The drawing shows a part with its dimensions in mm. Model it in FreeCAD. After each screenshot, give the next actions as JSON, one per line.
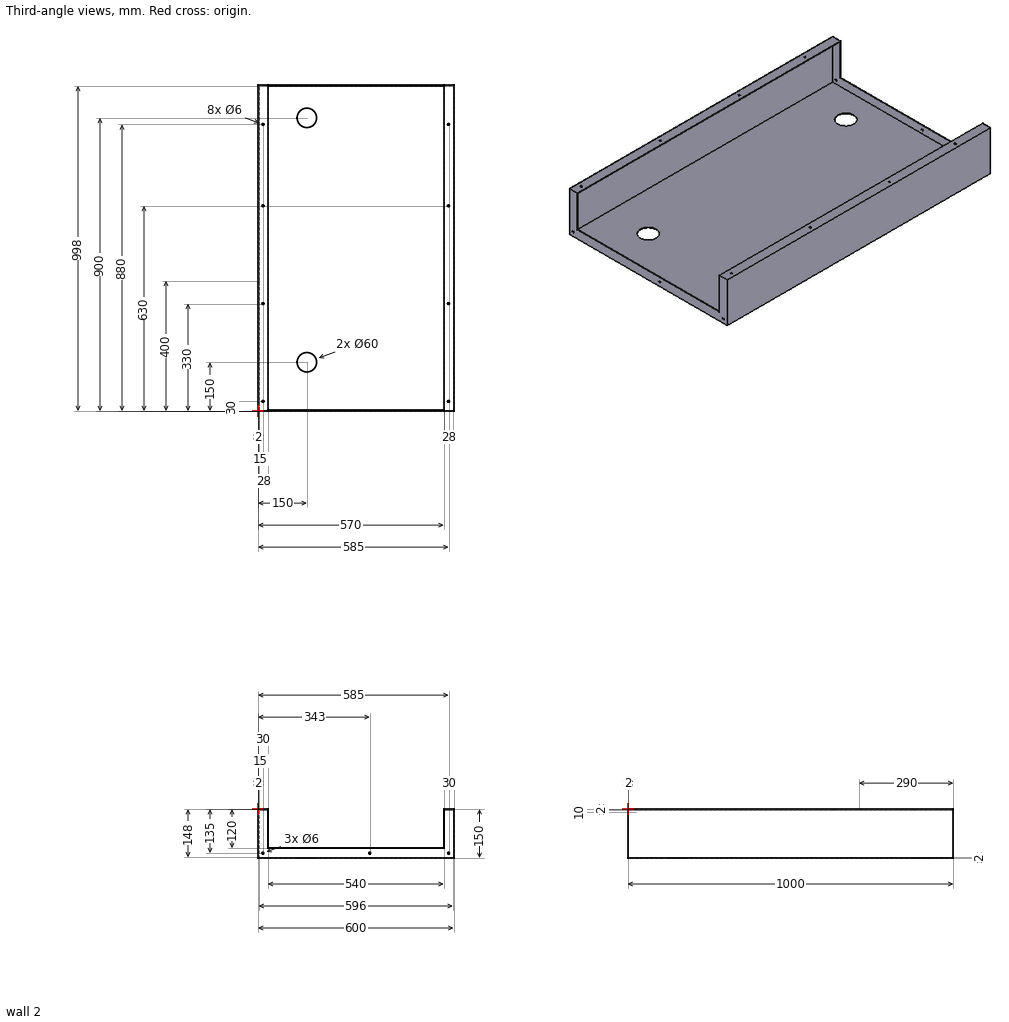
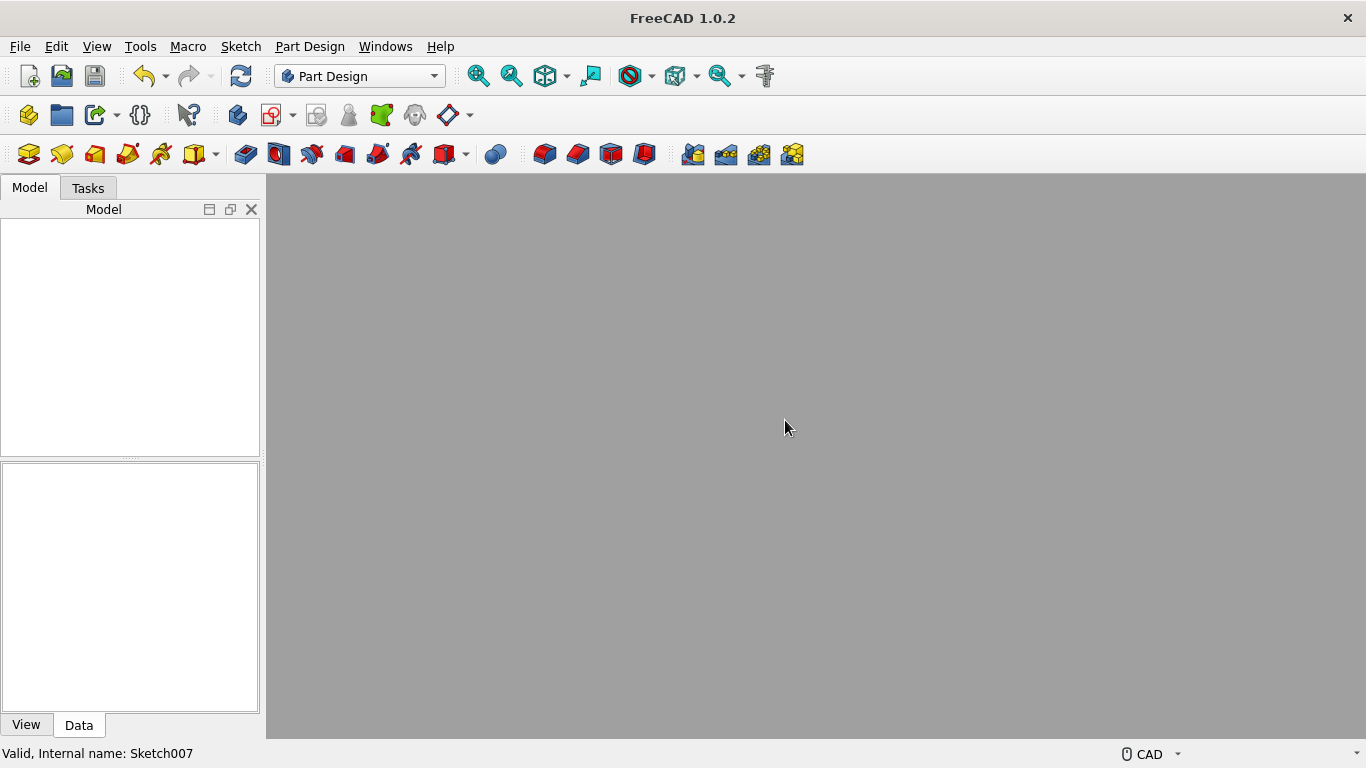
{"action": "left_click", "coordinate": [29, 76]}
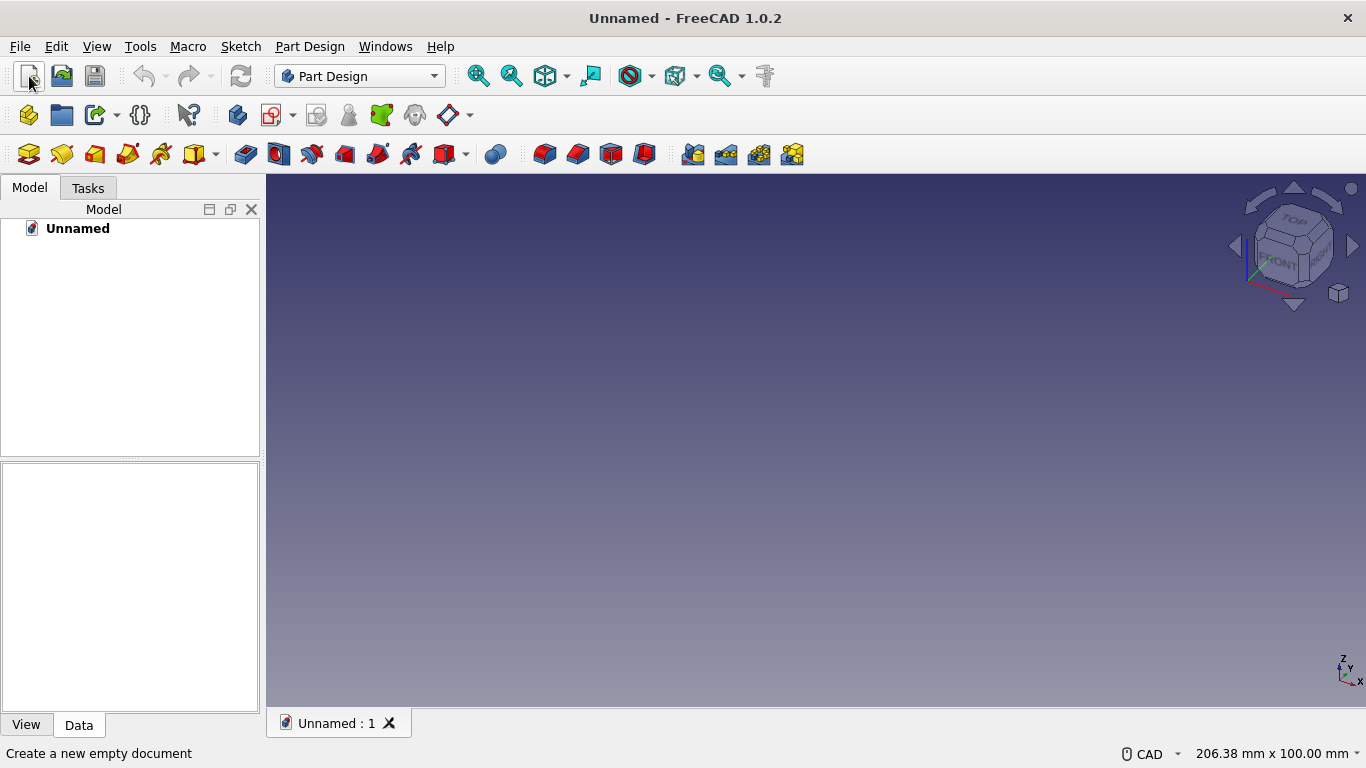
{"action": "left_click", "coordinate": [270, 116]}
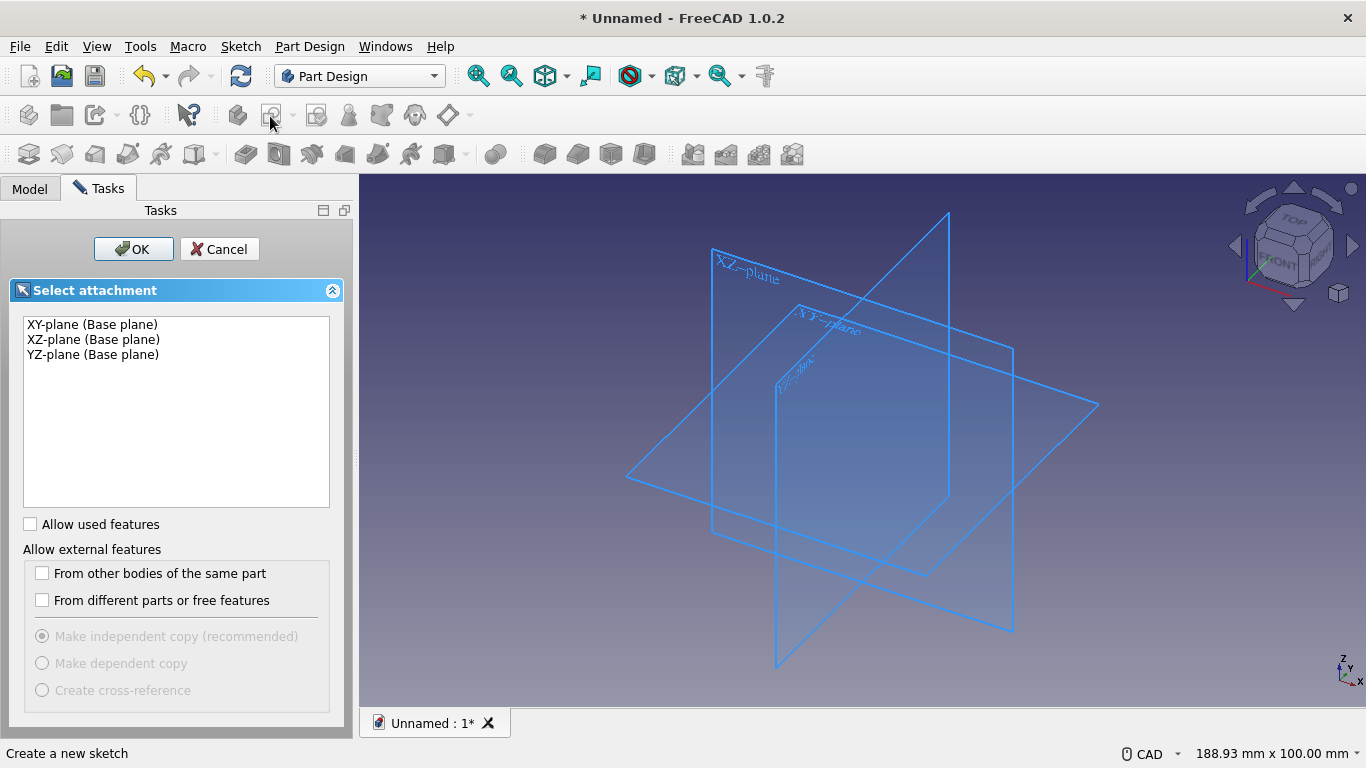
{"action": "left_click", "coordinate": [84, 340]}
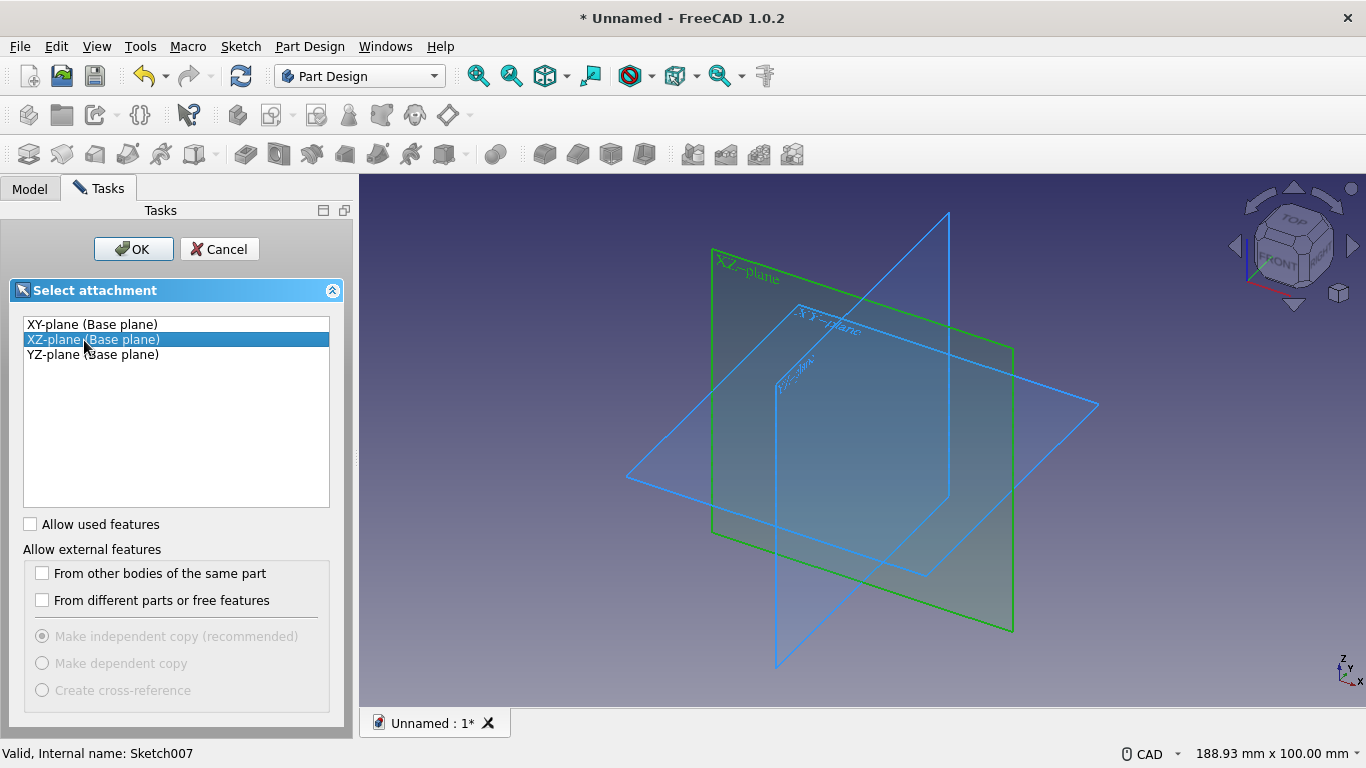
{"action": "left_click", "coordinate": [134, 249]}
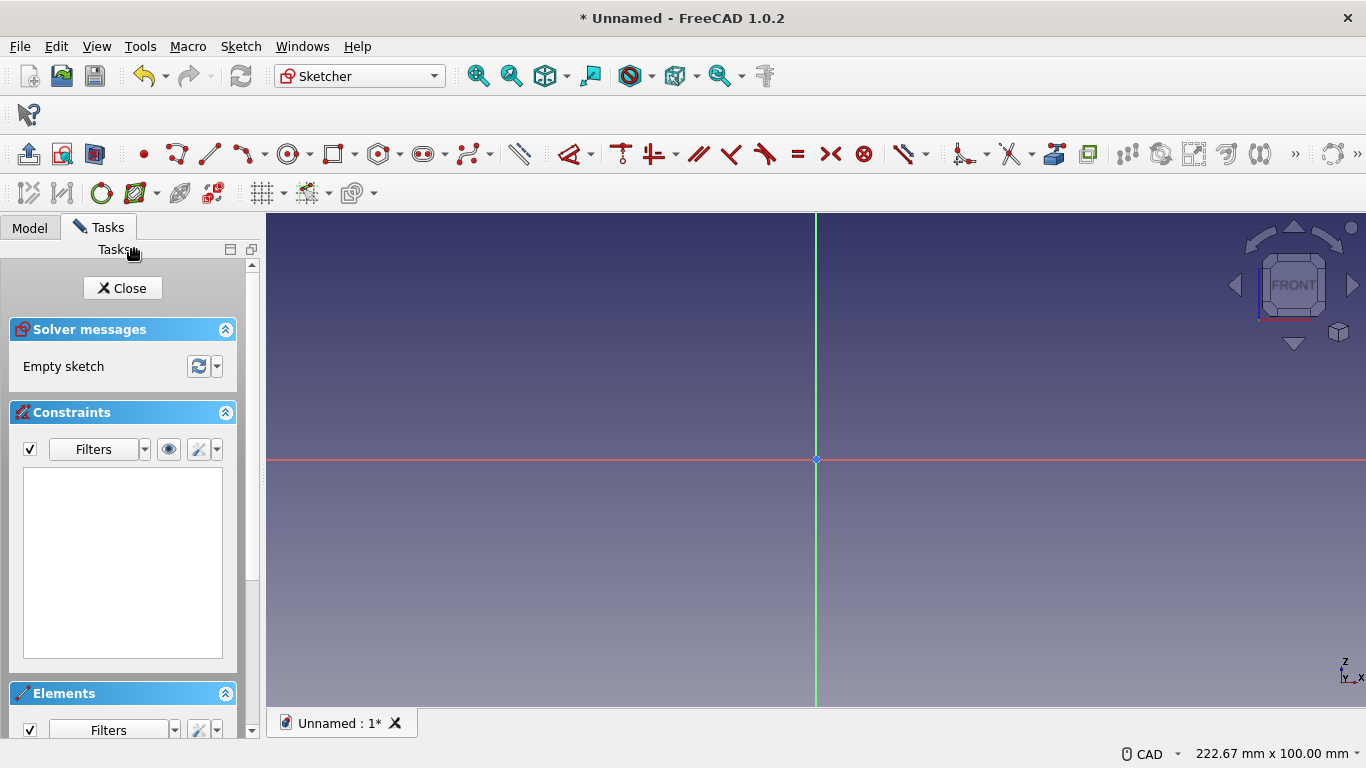
{"action": "scroll", "coordinate": [355, 366], "scroll_direction": "down", "scroll_amount": 8}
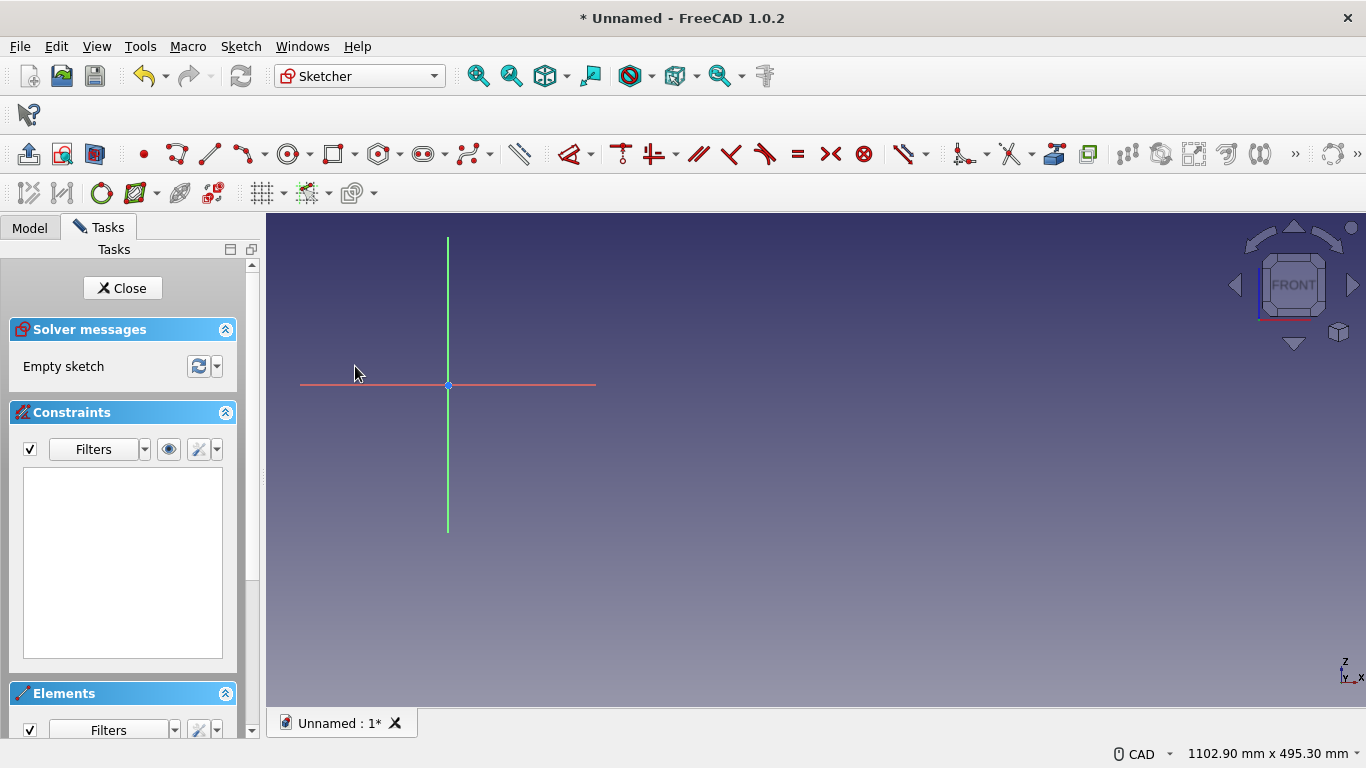
{"action": "left_click", "coordinate": [332, 154]}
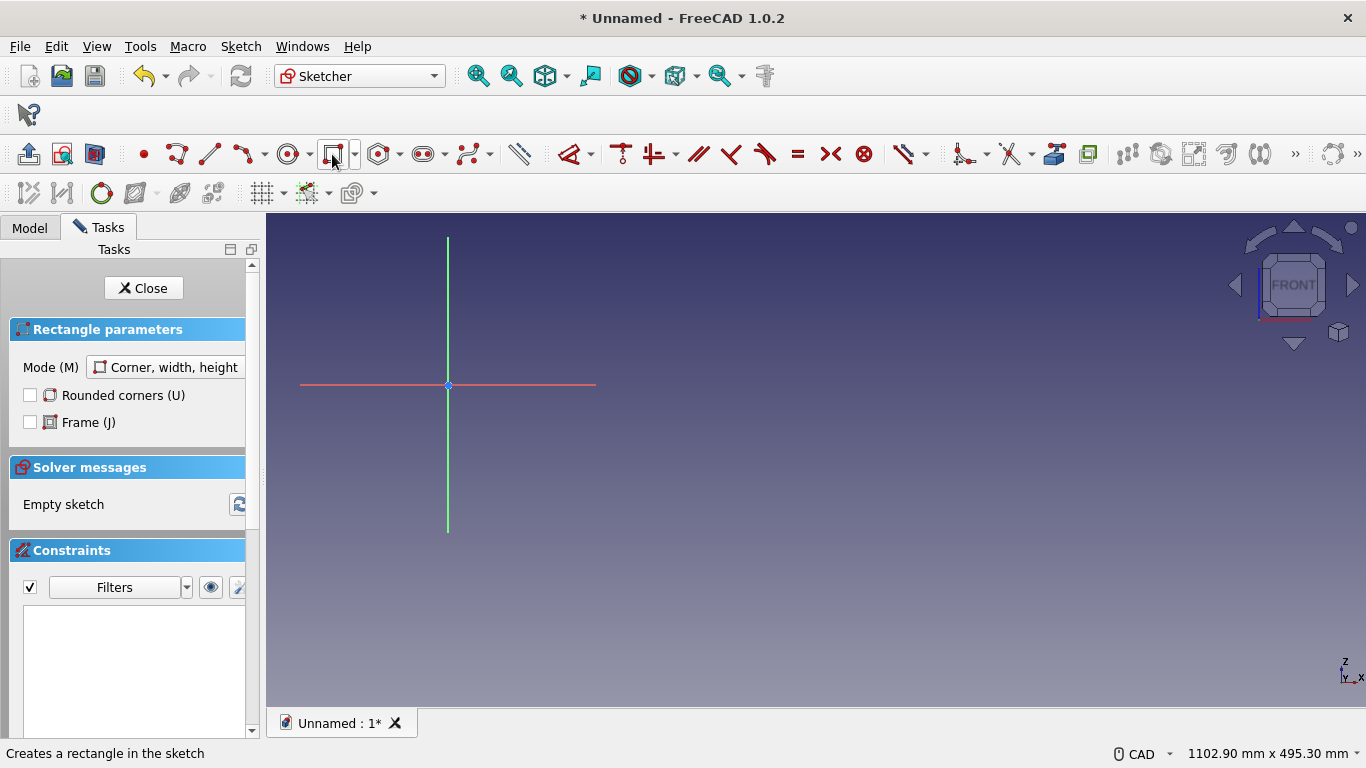
{"action": "left_click", "coordinate": [448, 385]}
{"action": "mouse_move", "coordinate": [1047, 535]}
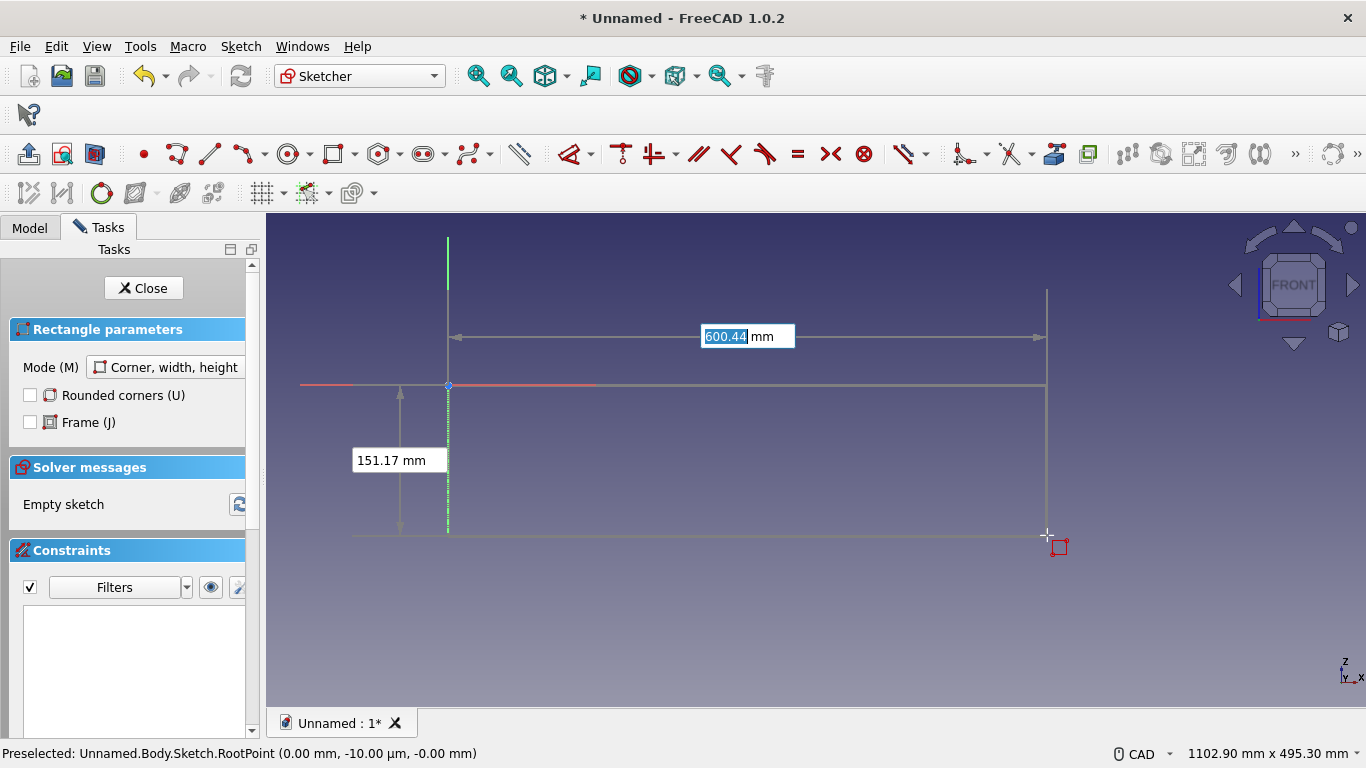
{"action": "type", "text": "600"}
{"action": "key", "text": "Tab"}
{"action": "type", "text": "150"}
{"action": "key", "text": "Return"}
{"action": "key", "text": "Escape"}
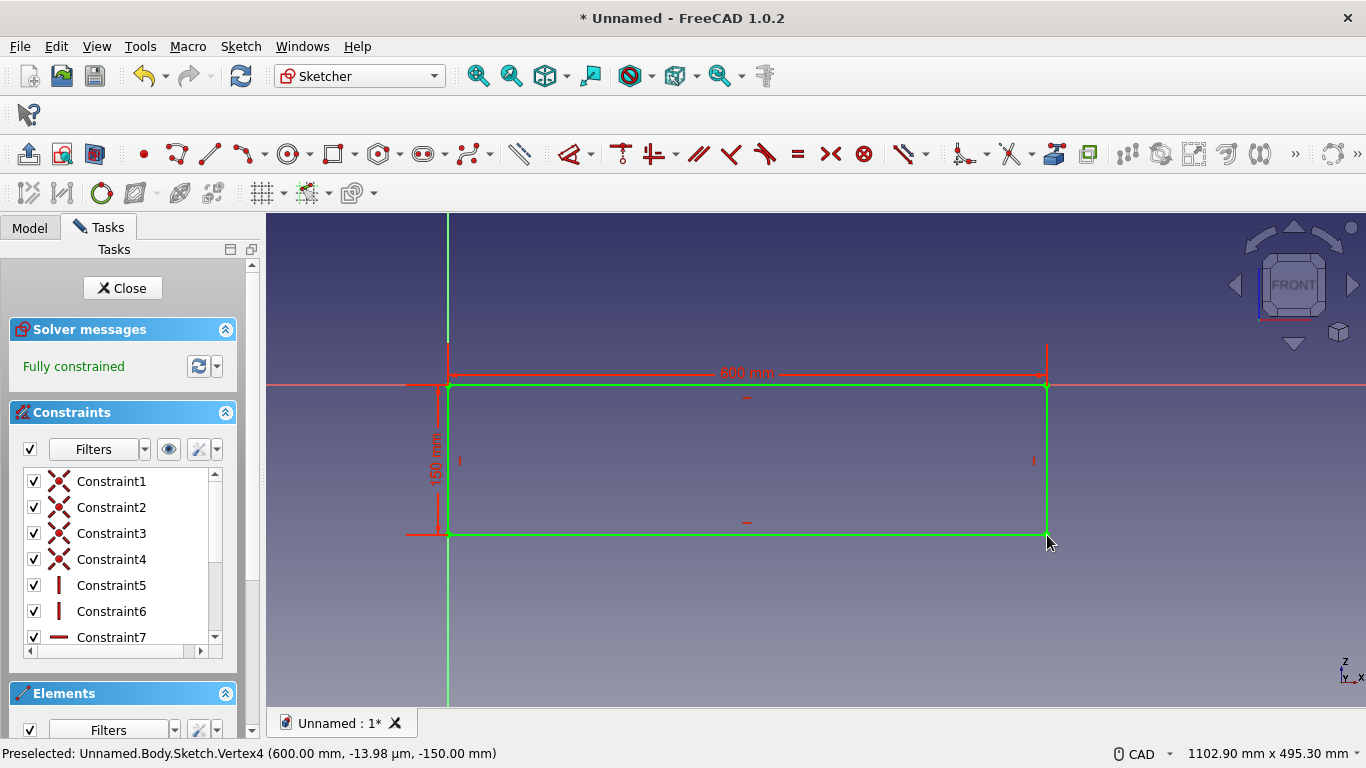
{"action": "left_click", "coordinate": [123, 288]}